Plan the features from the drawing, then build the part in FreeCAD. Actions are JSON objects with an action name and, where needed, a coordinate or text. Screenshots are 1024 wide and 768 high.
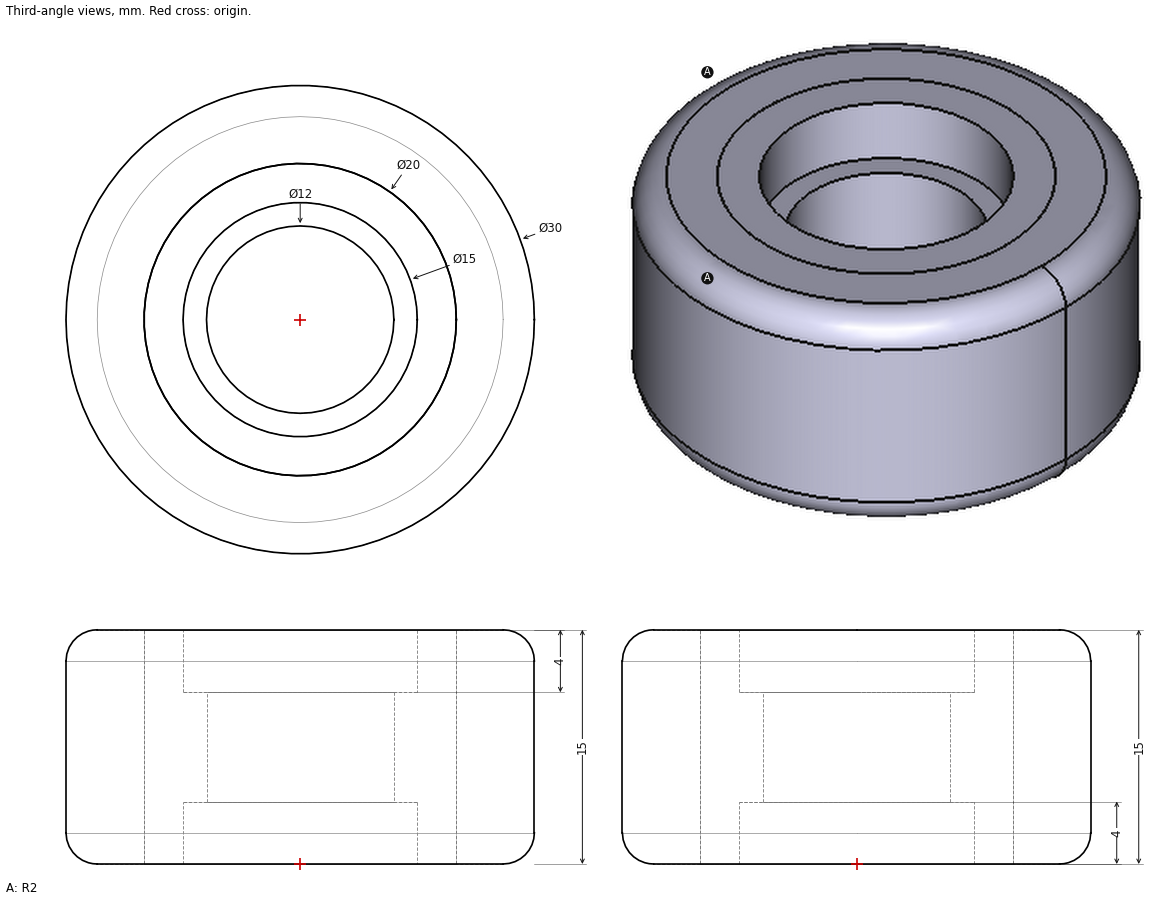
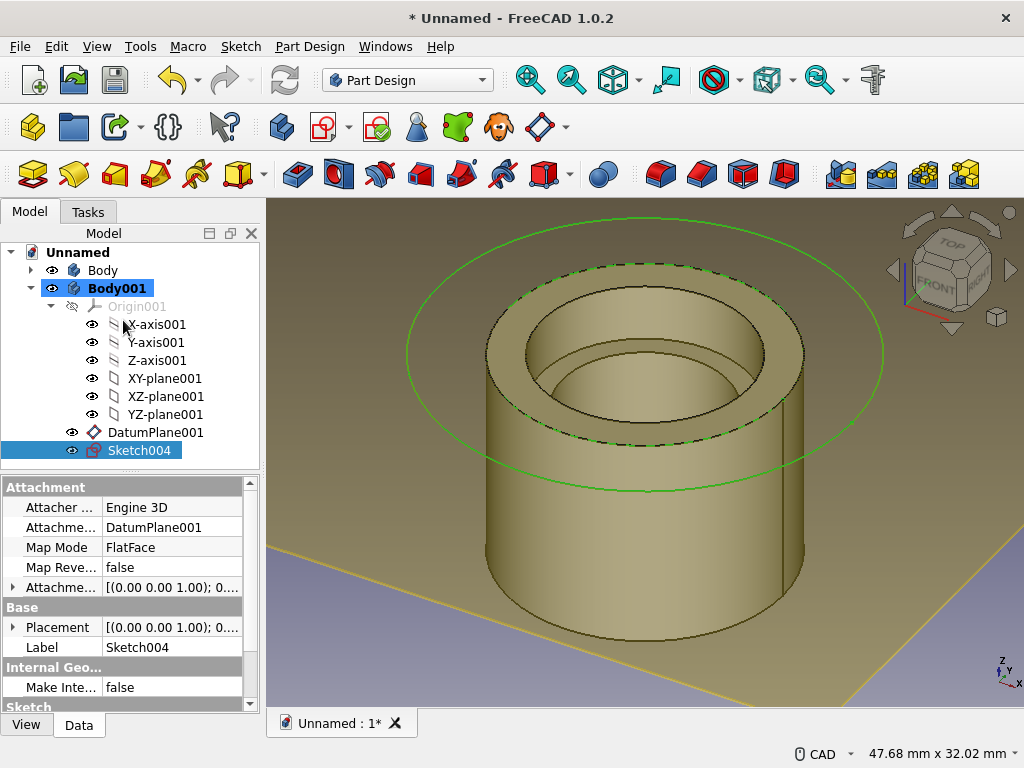
{"action": "left_click", "coordinate": [33, 174]}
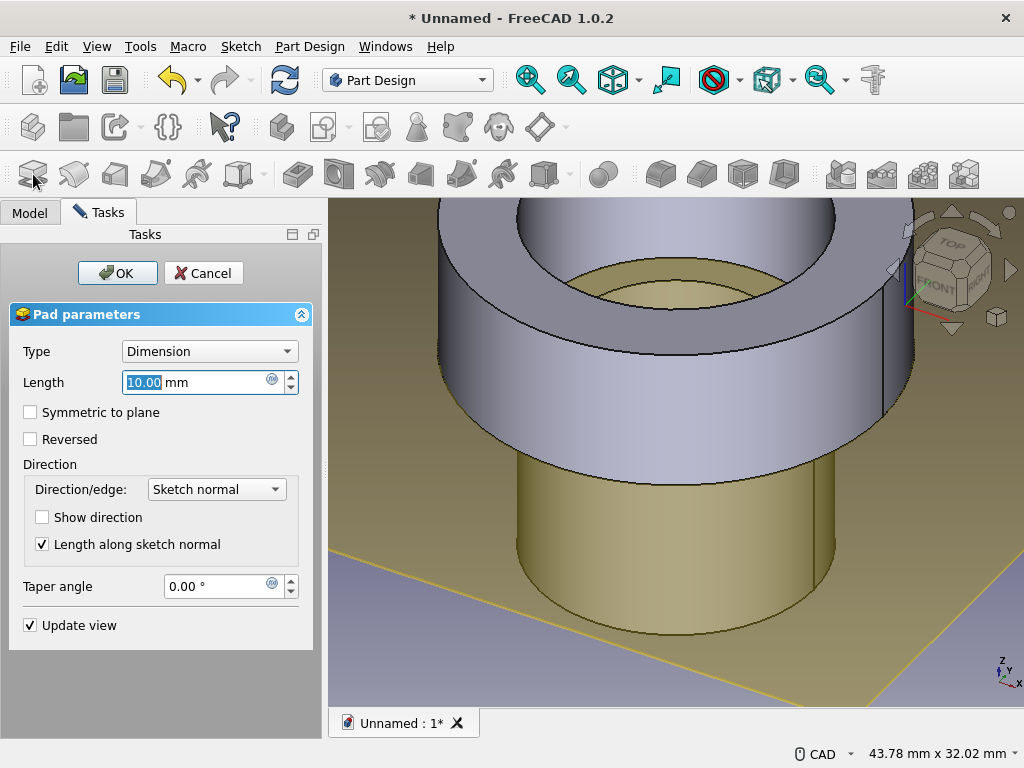
{"action": "type", "text": "15"}
{"action": "key", "text": "Tab"}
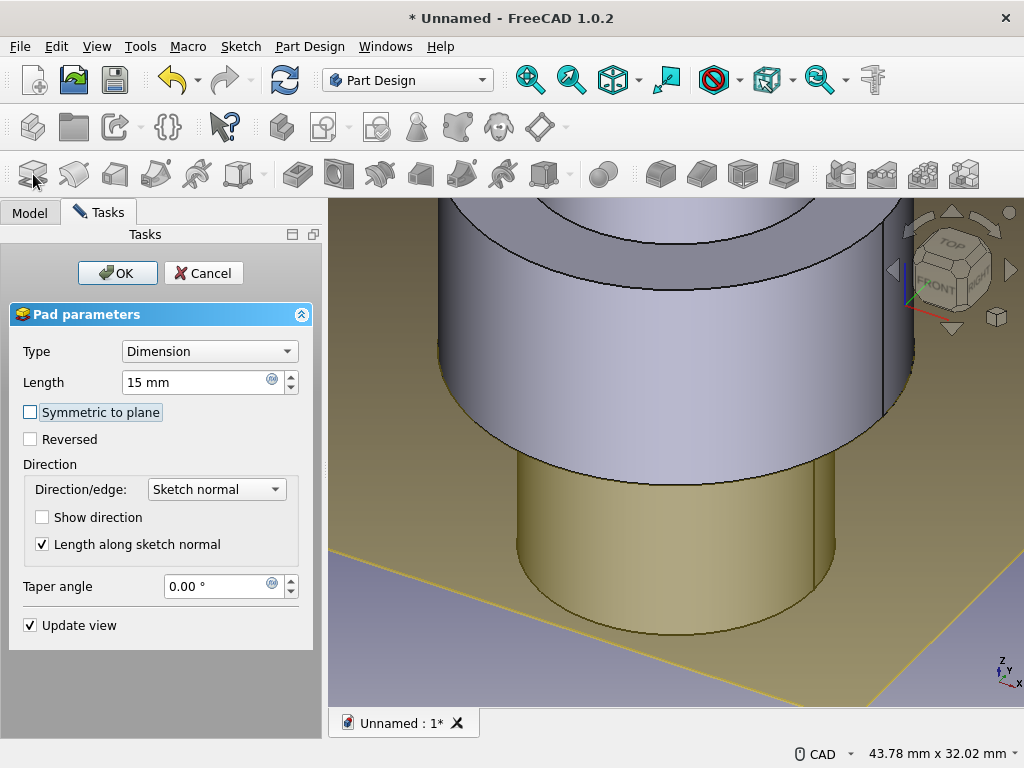
{"action": "left_click", "coordinate": [31, 439]}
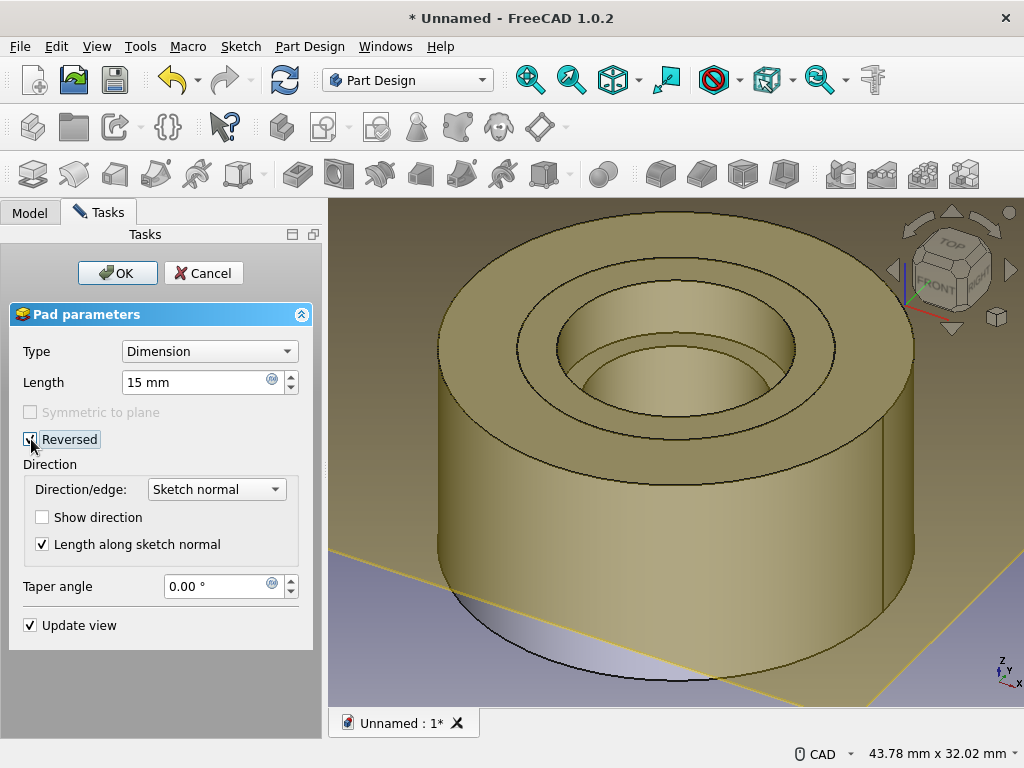
{"action": "left_click", "coordinate": [118, 273]}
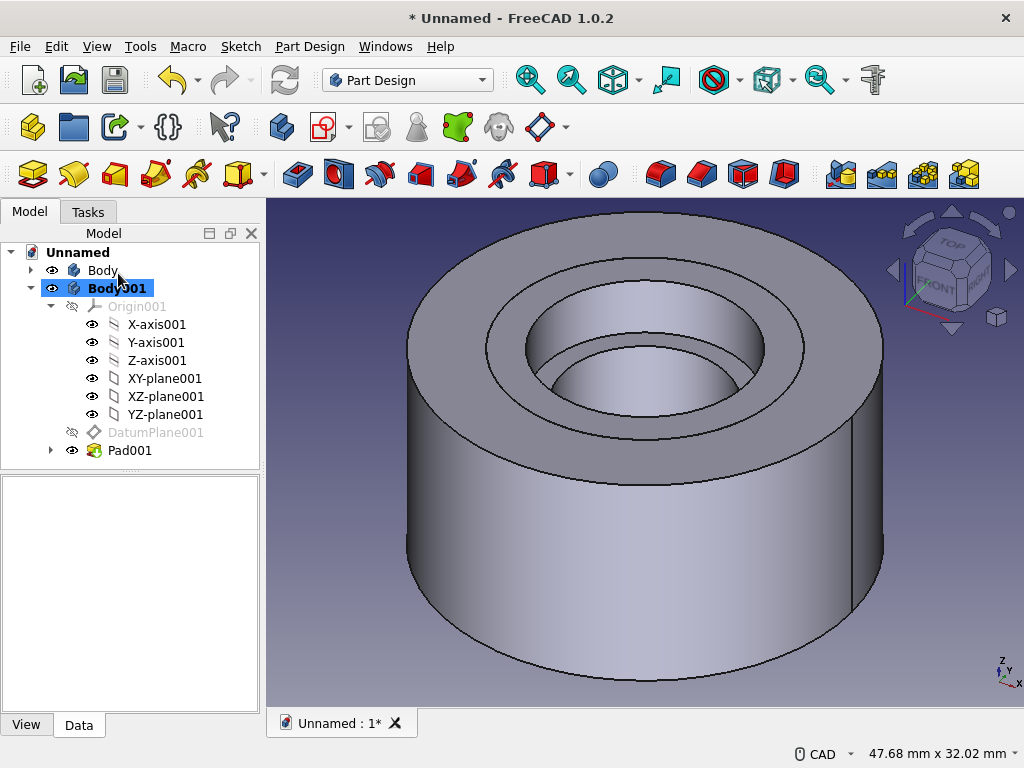
{"action": "left_click", "coordinate": [531, 80]}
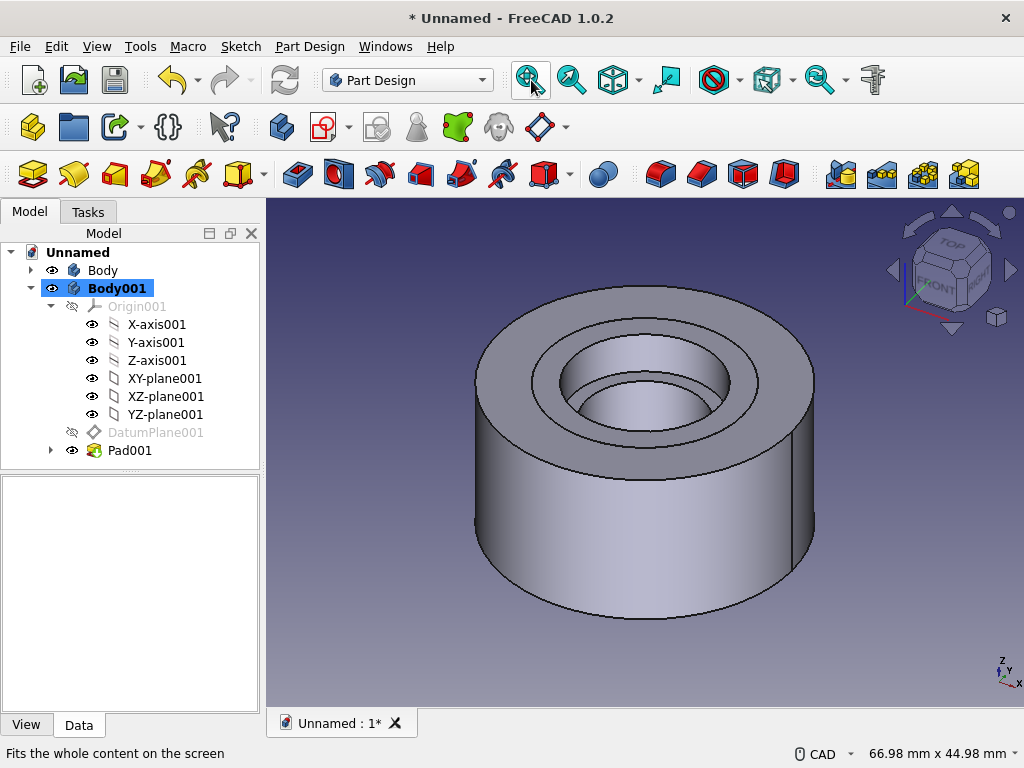
{"action": "left_click", "coordinate": [476, 392]}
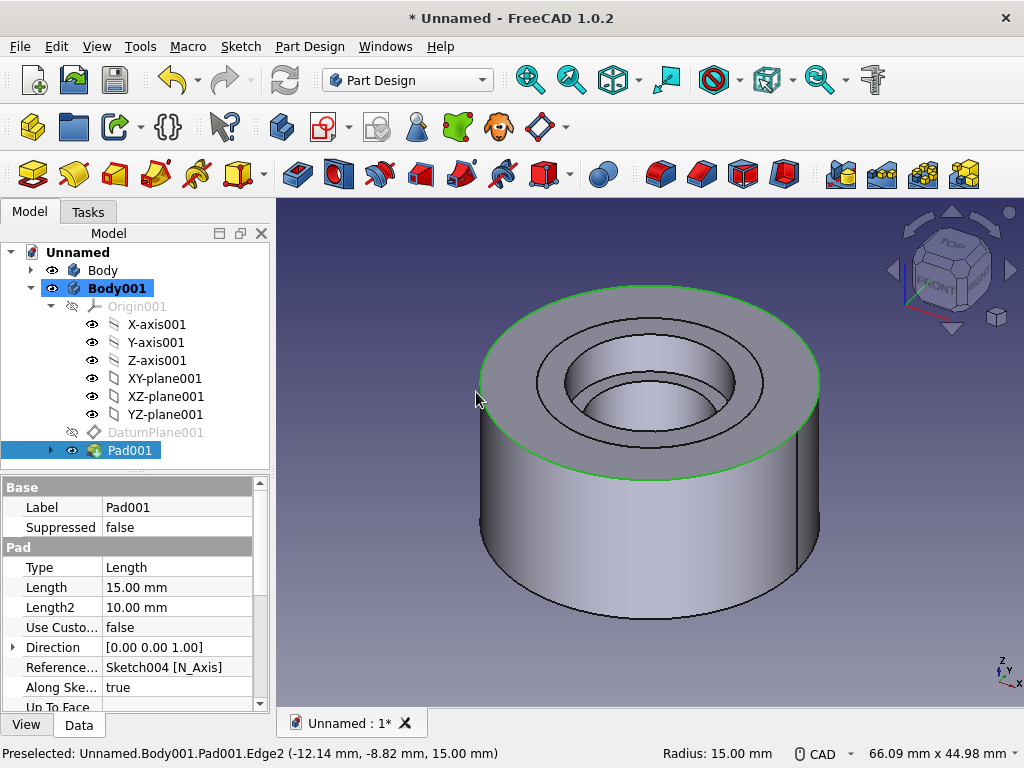
{"action": "key", "text": "0"}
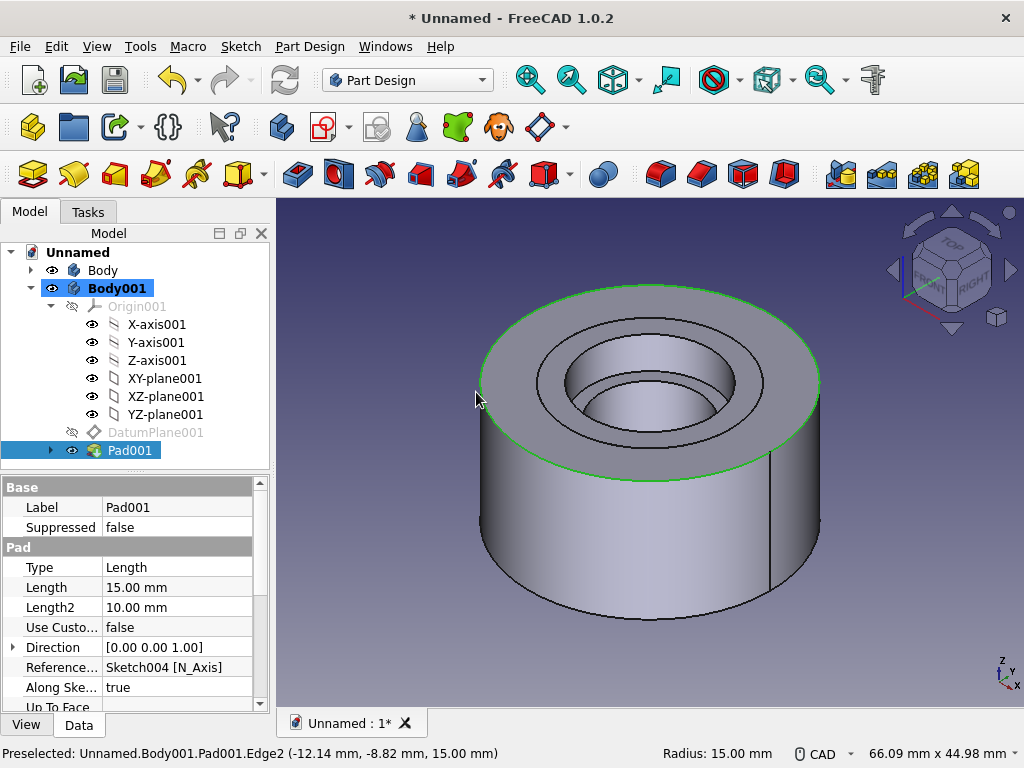
{"action": "key", "text": "2"}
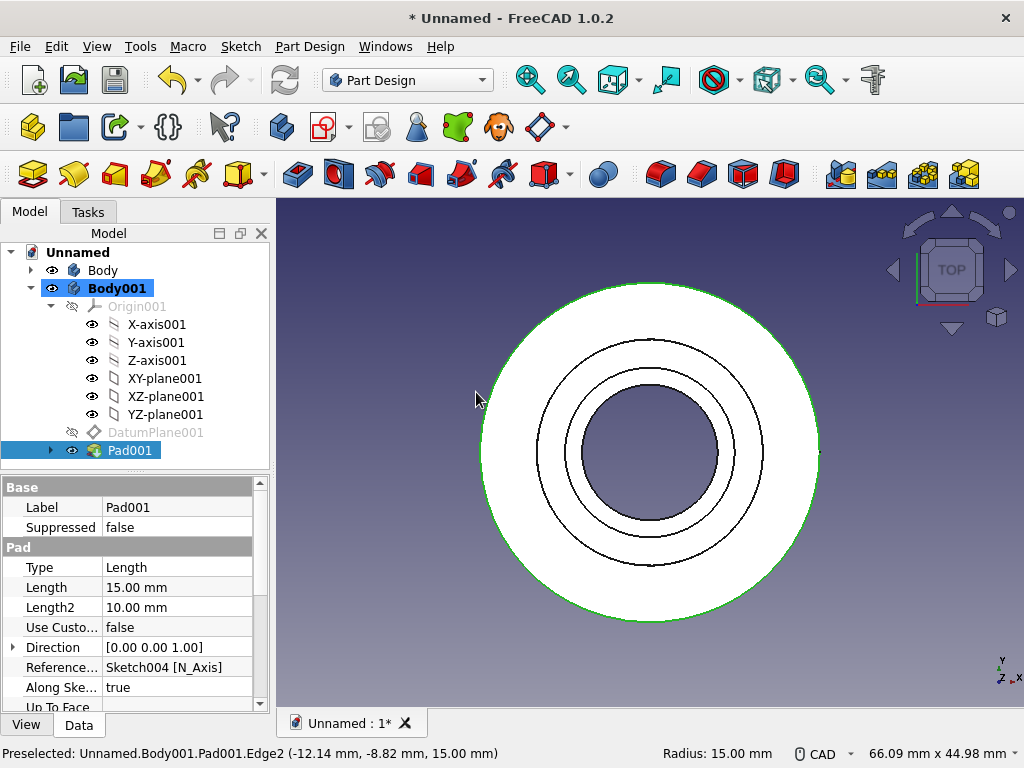
{"action": "key", "text": "1"}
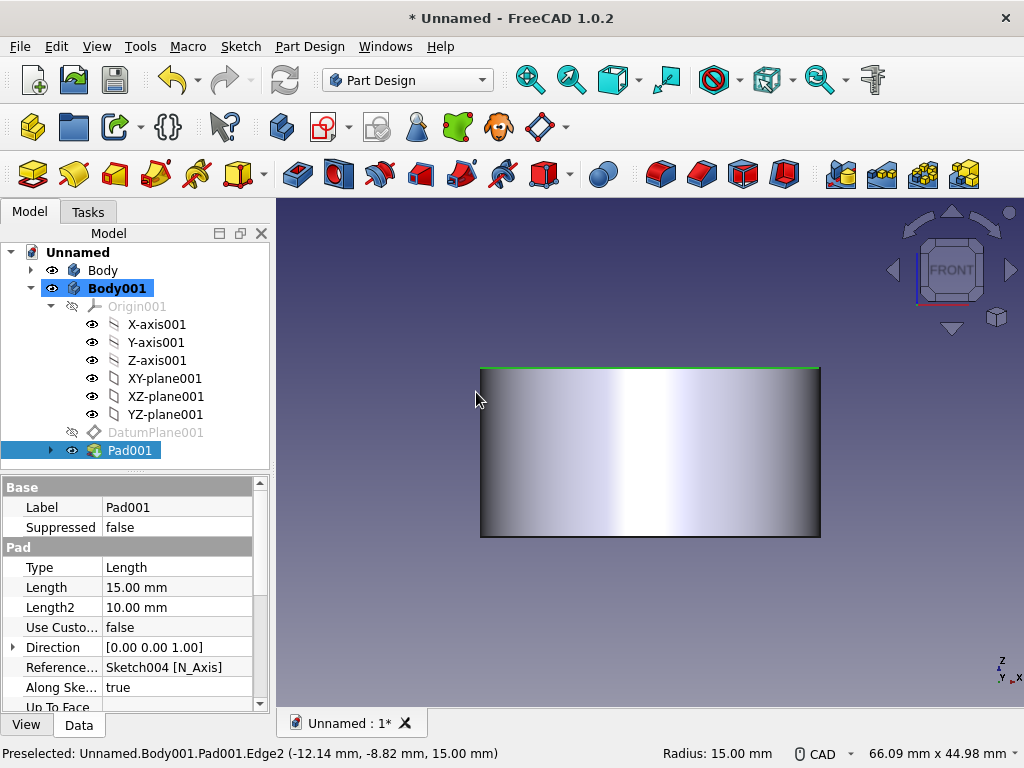
{"action": "left_click", "coordinate": [513, 536], "text": "ctrl"}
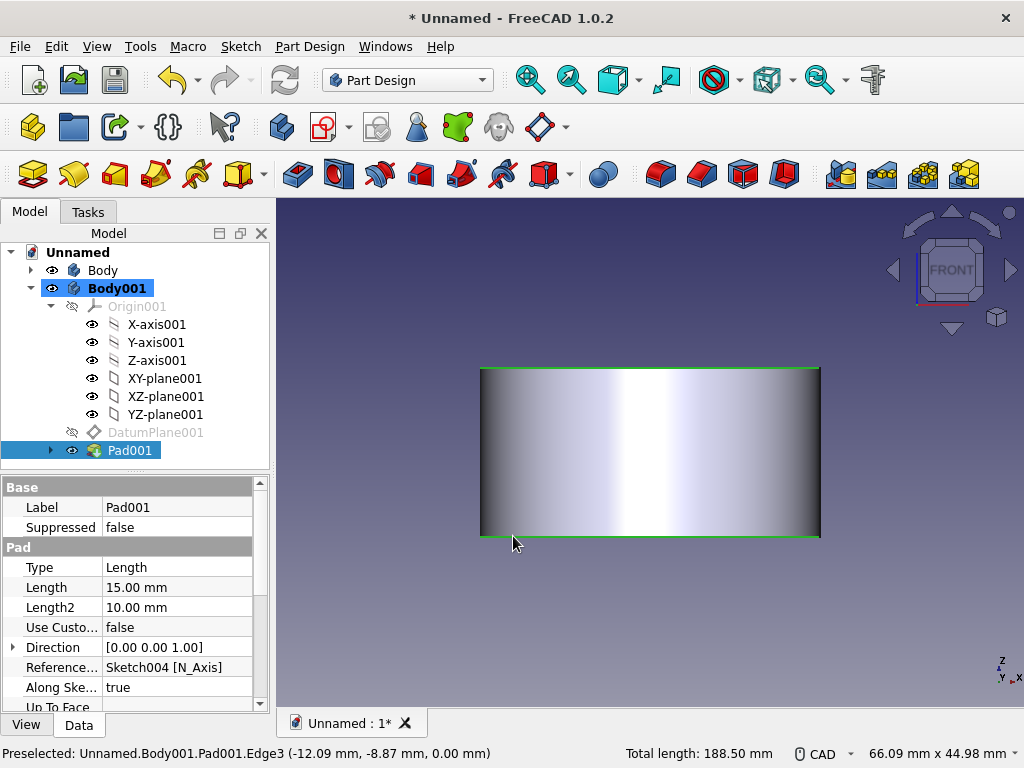
{"action": "left_click", "coordinate": [661, 174]}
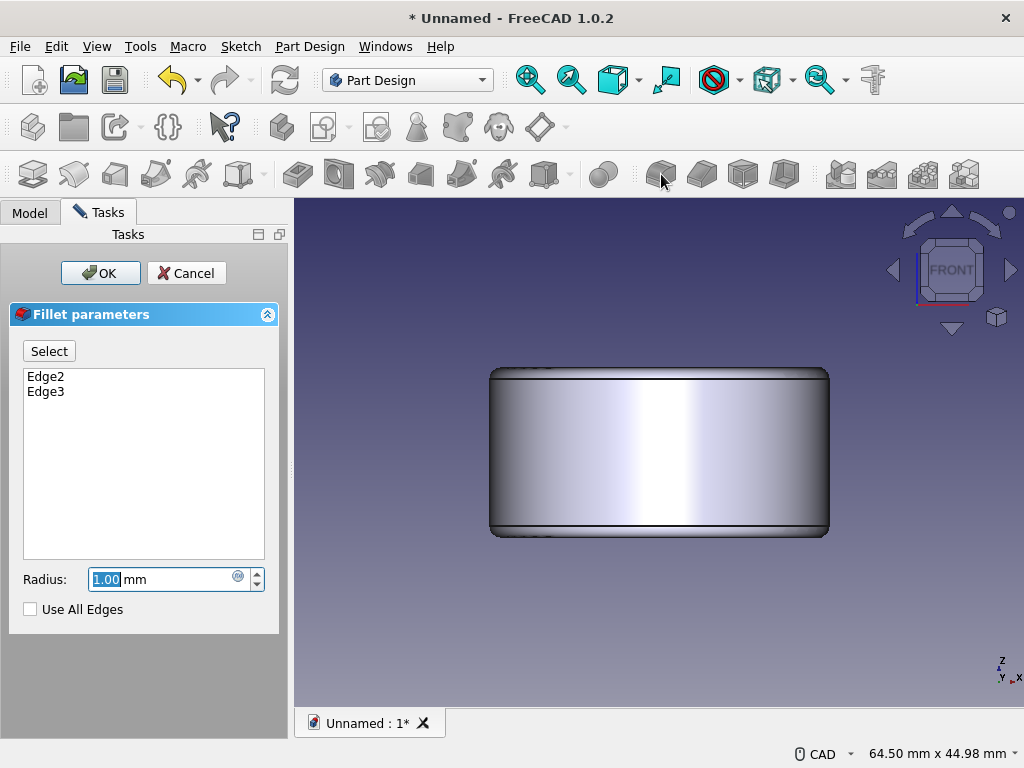
{"action": "type", "text": "2"}
{"action": "key", "text": "Tab"}